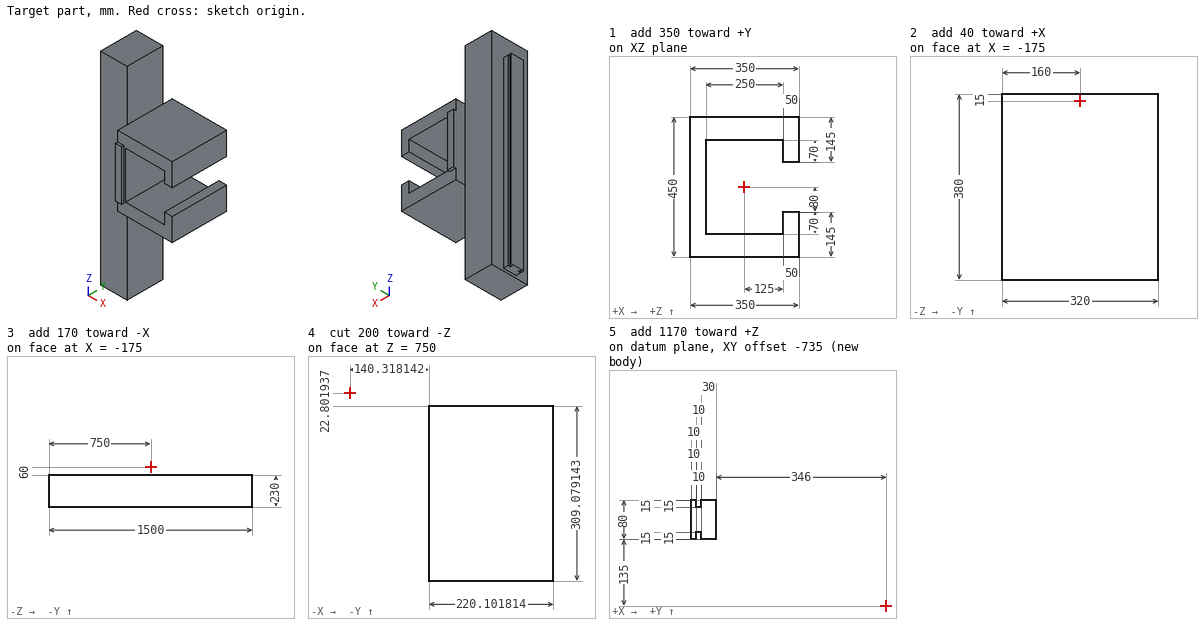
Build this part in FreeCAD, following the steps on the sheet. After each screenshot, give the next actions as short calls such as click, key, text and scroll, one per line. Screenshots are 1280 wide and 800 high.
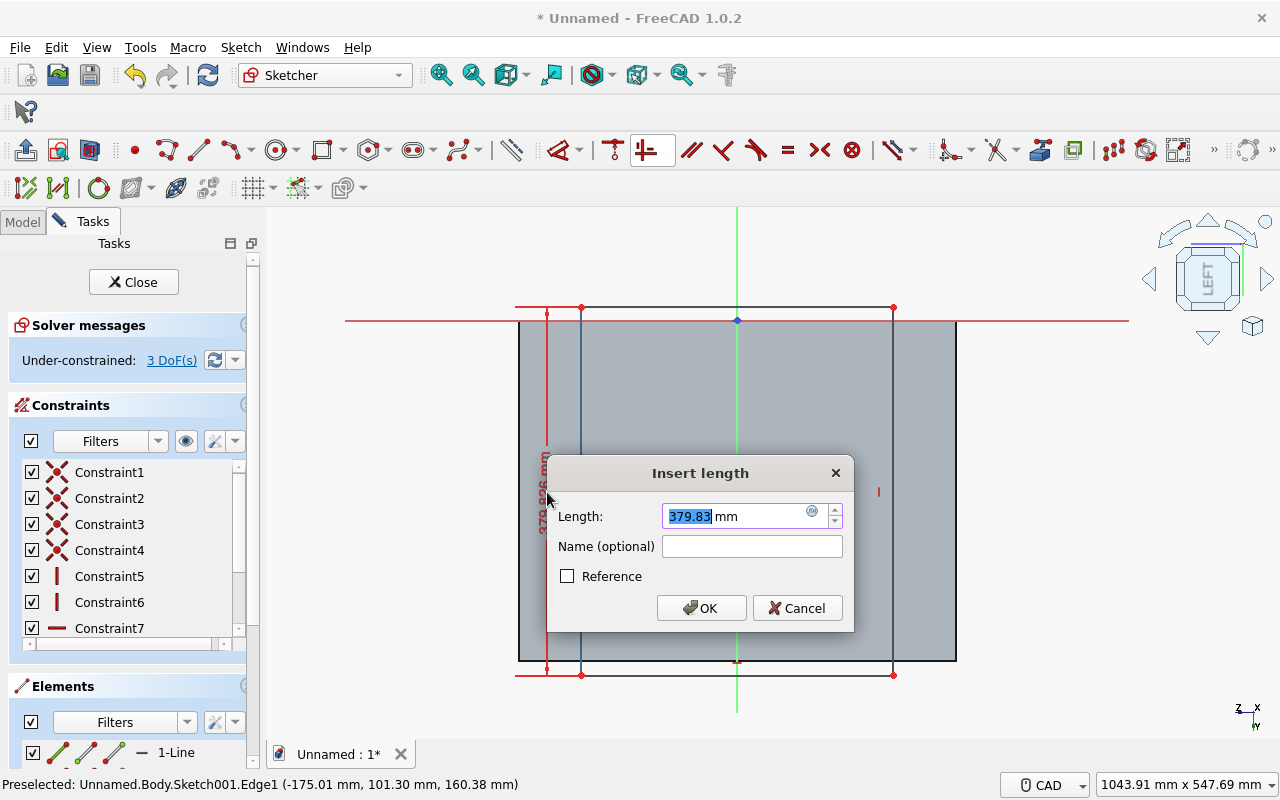
text(380)
key(Return)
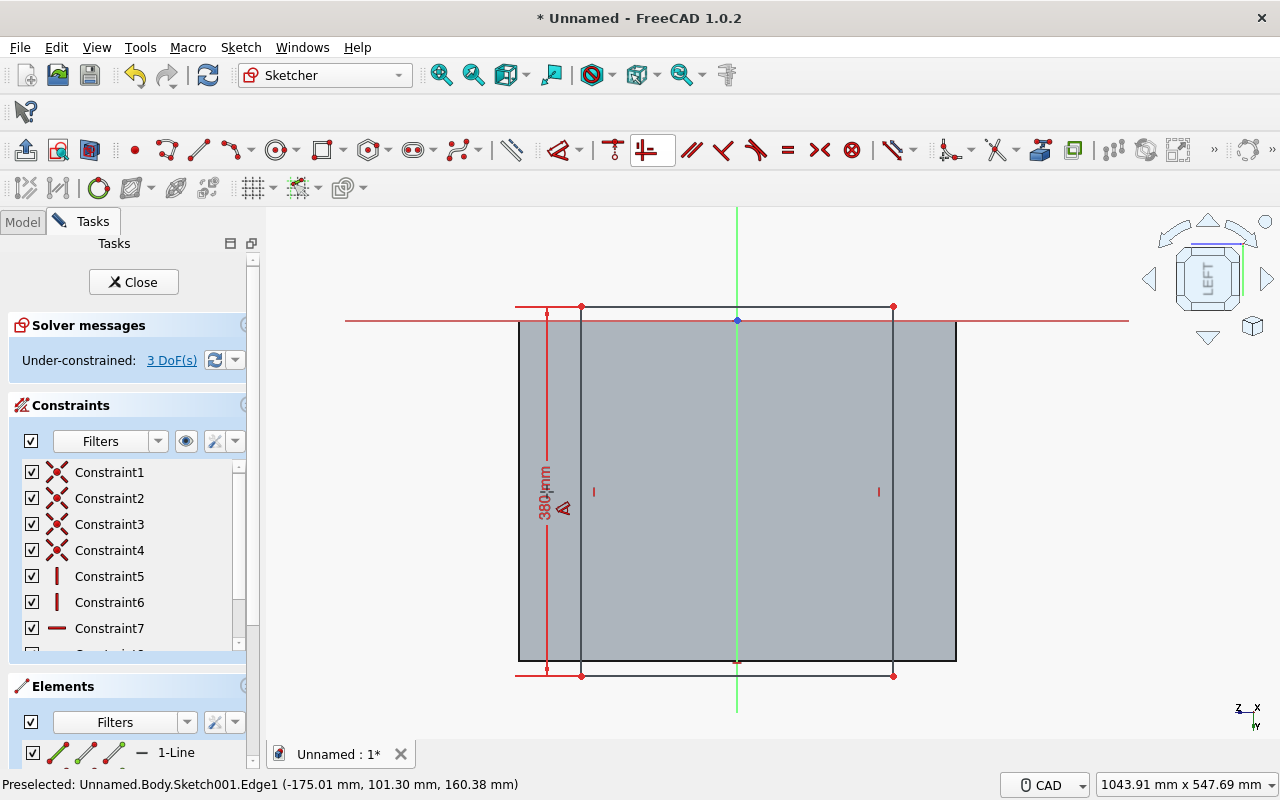
click(675, 676)
click(666, 710)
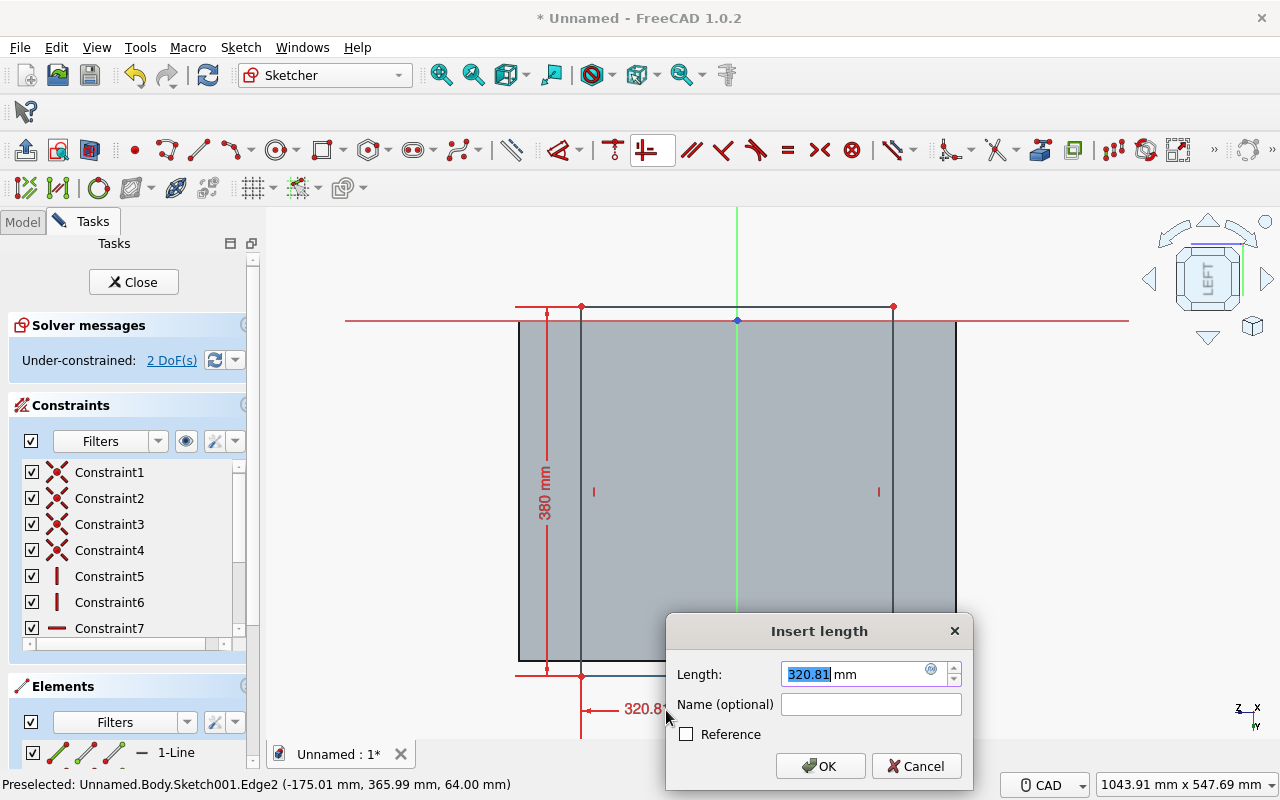
text(320)
key(Return)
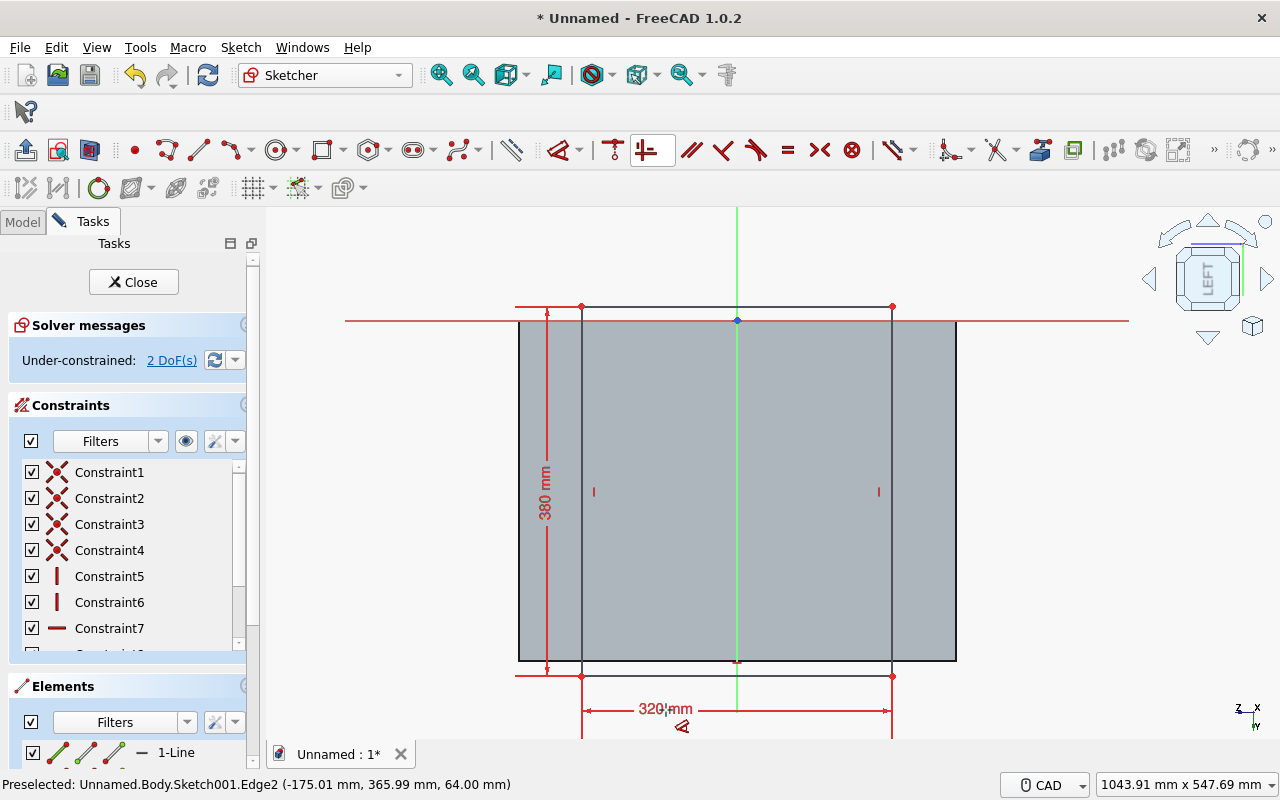
scroll(582, 307, up, 6)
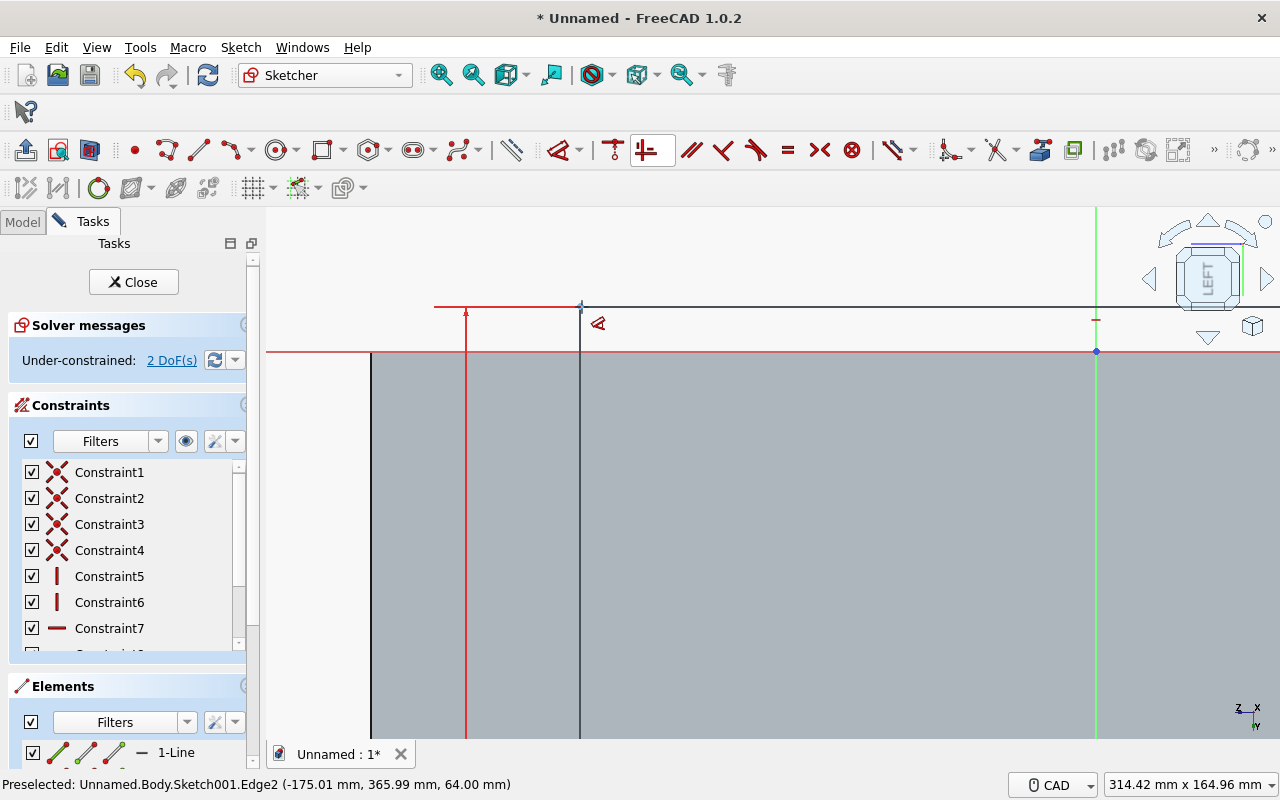
click(580, 307)
click(546, 329)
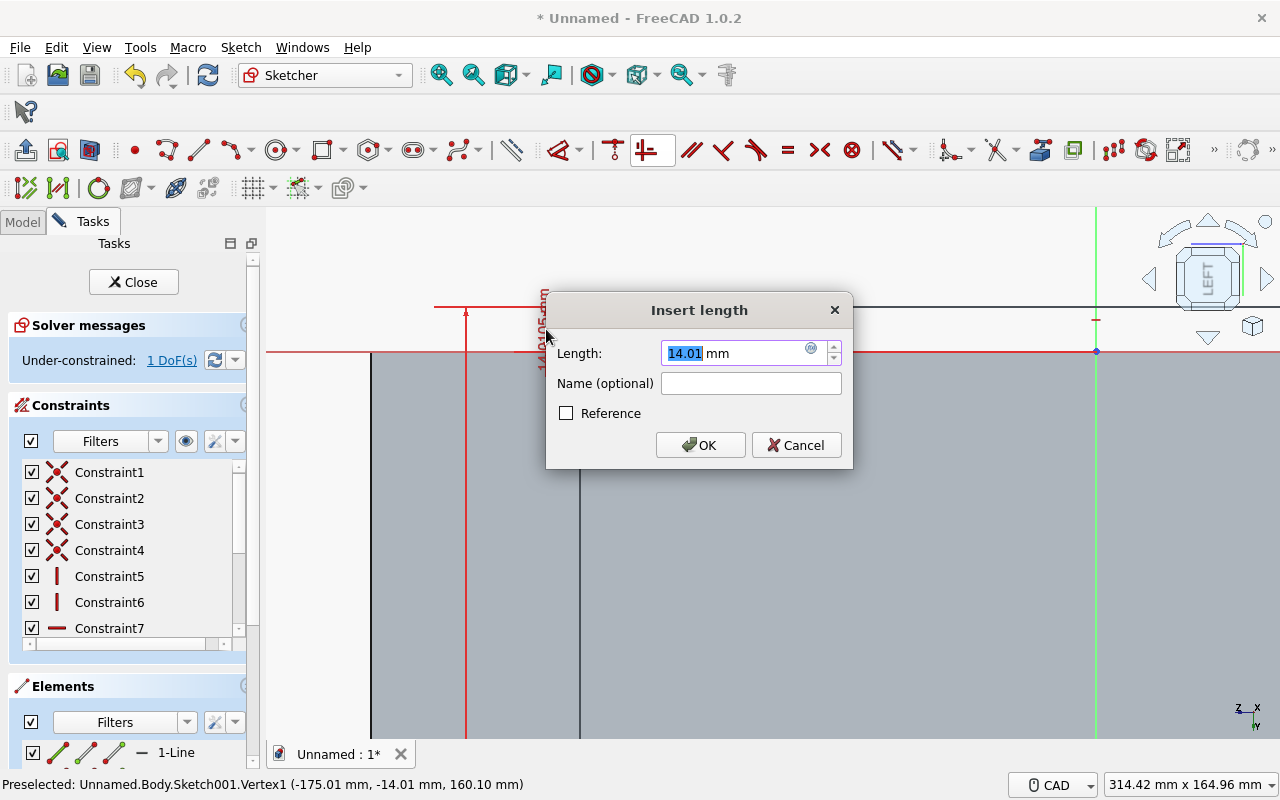
text(15)
key(Return)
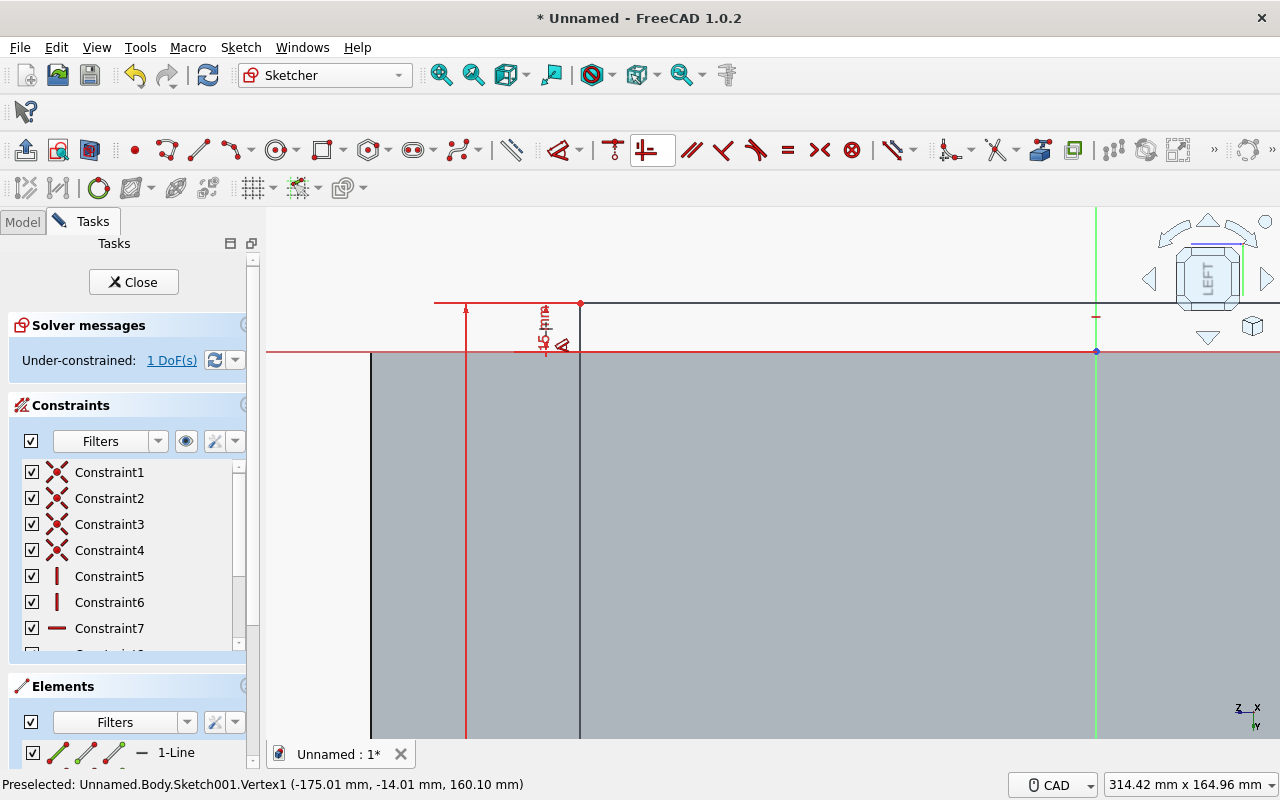
scroll(536, 282, down, 6)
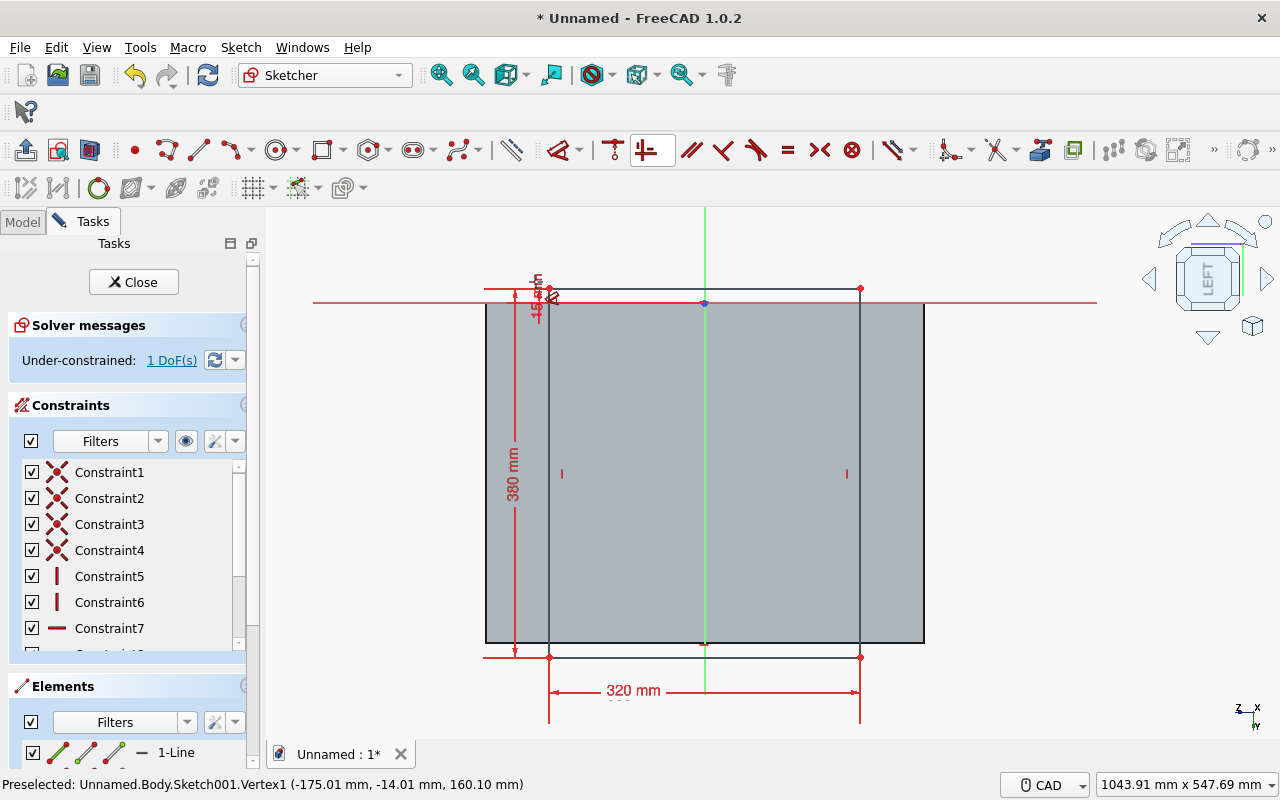
click(549, 289)
click(627, 255)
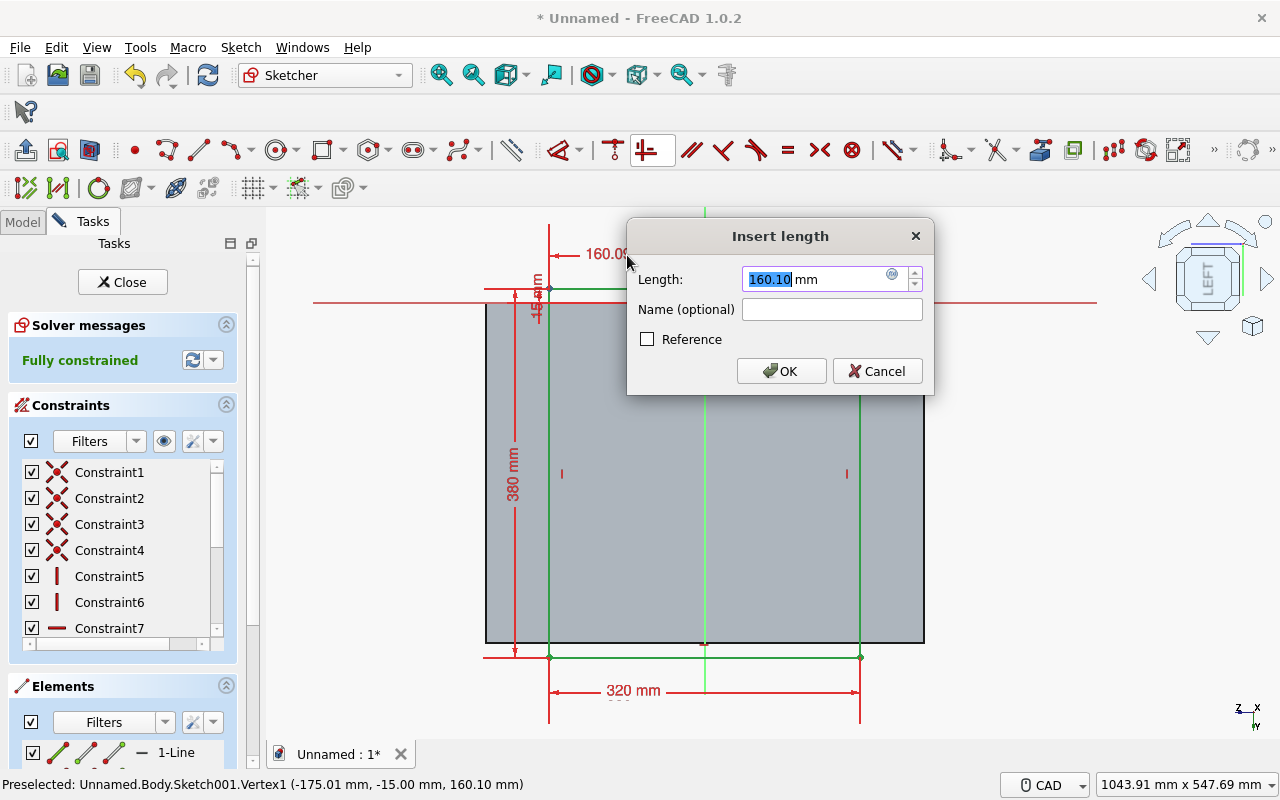
text(160)
key(Return)
key(Escape)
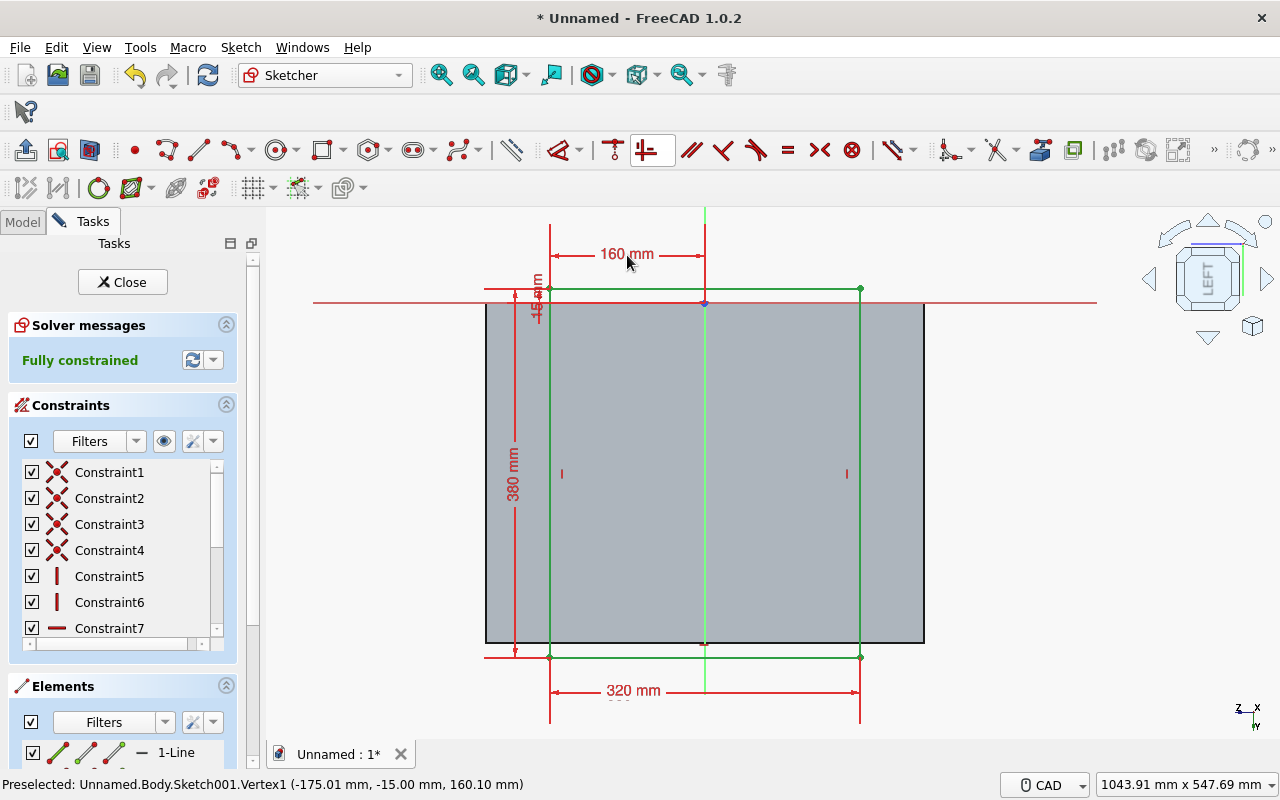
click(123, 282)